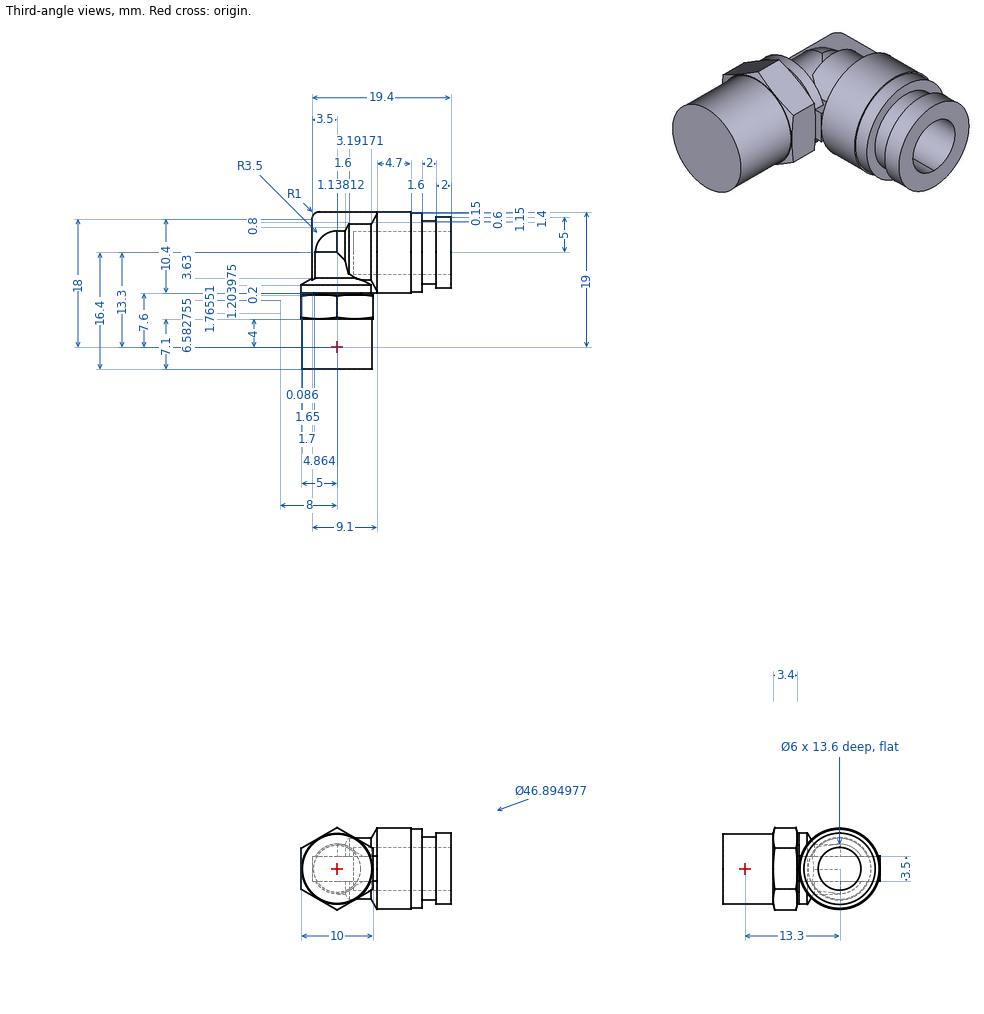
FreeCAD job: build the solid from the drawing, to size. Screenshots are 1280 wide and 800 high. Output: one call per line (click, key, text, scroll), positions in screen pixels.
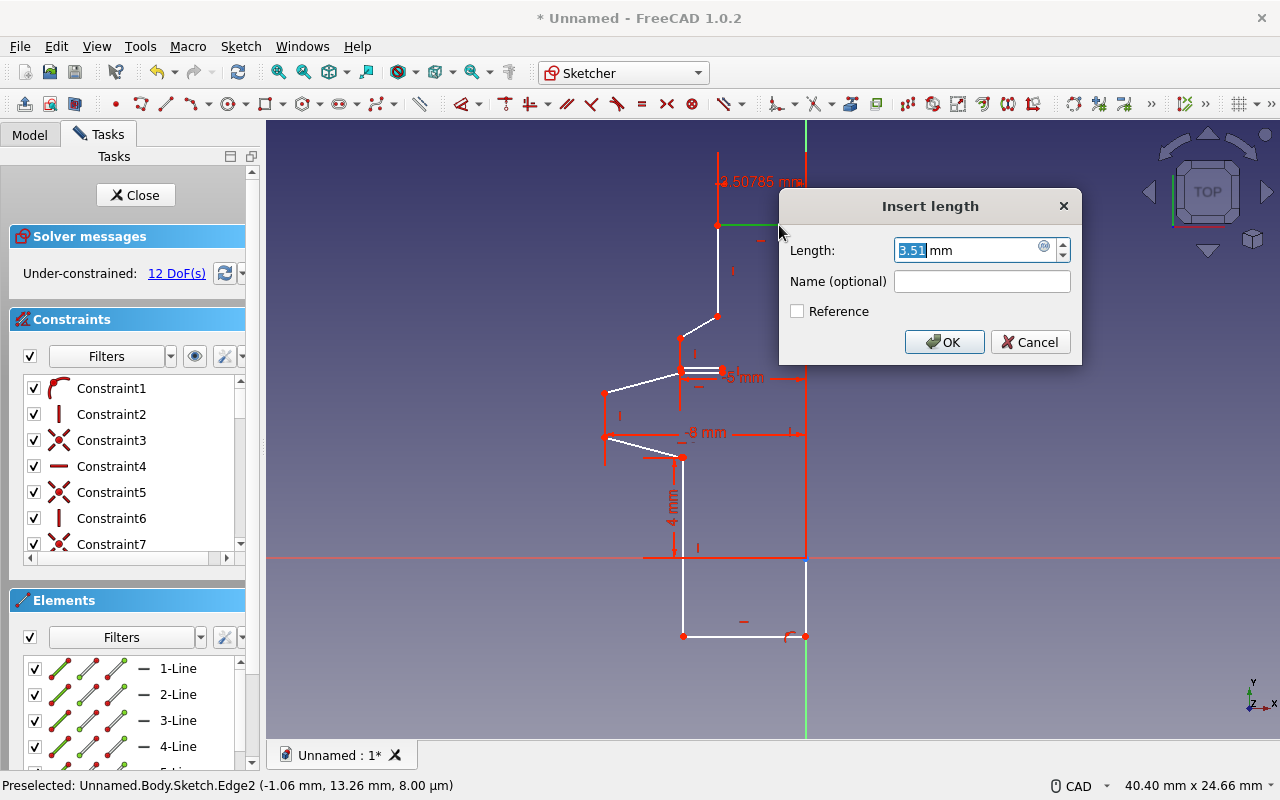
text(3.5)
key(Return)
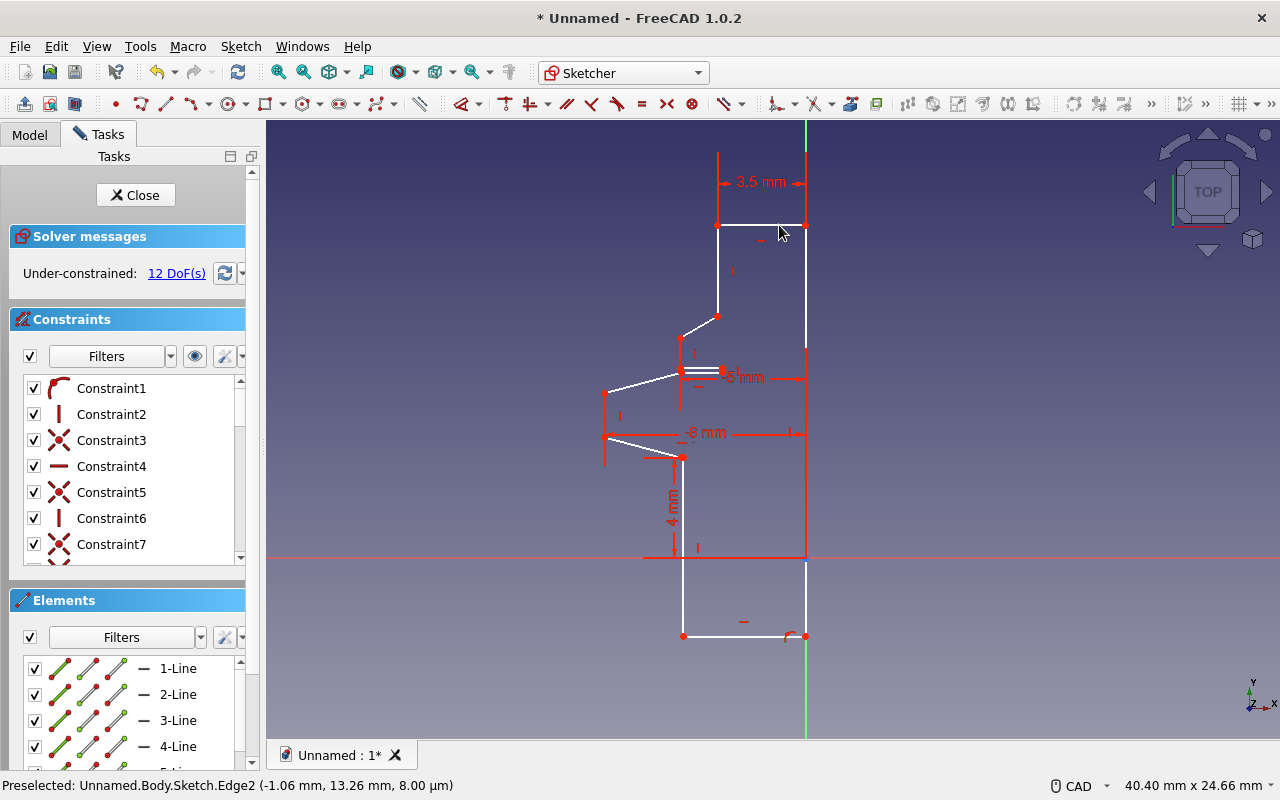
scroll(693, 368, up, 6)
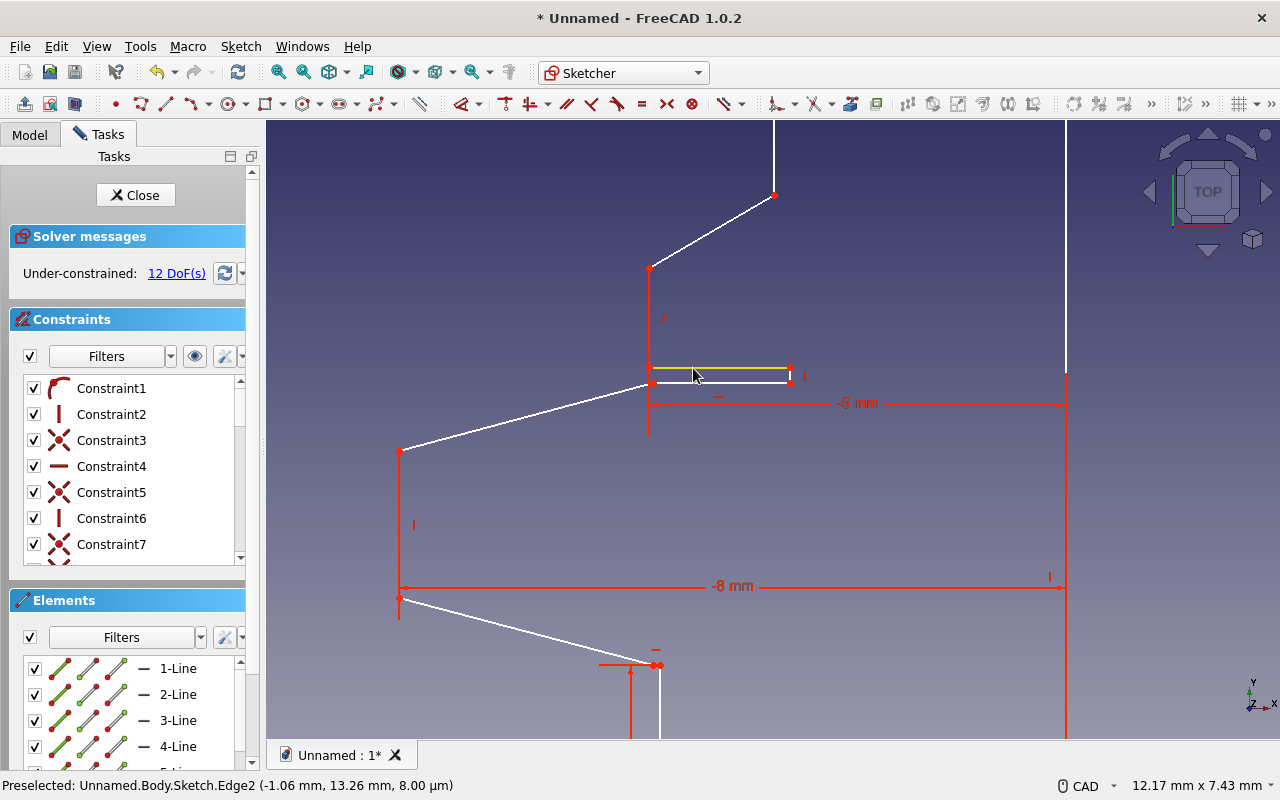
click(692, 368)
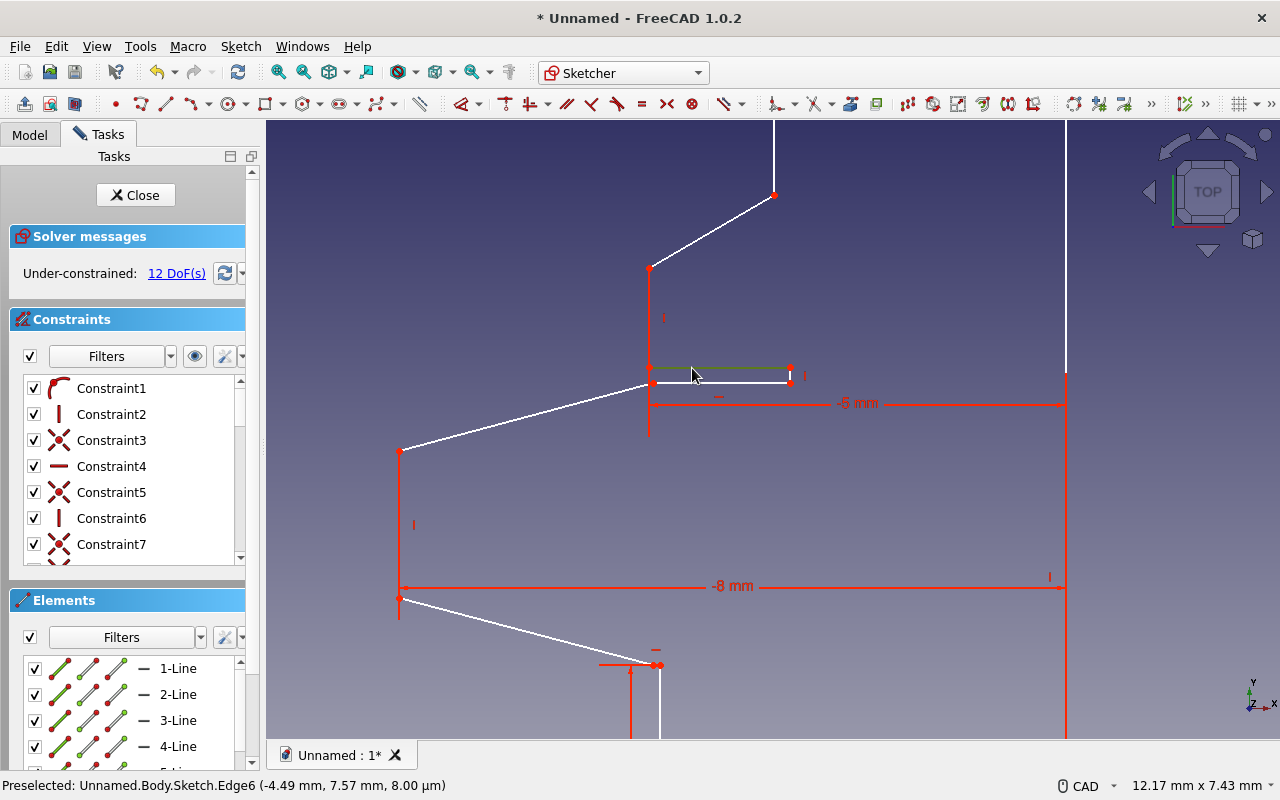
key(l)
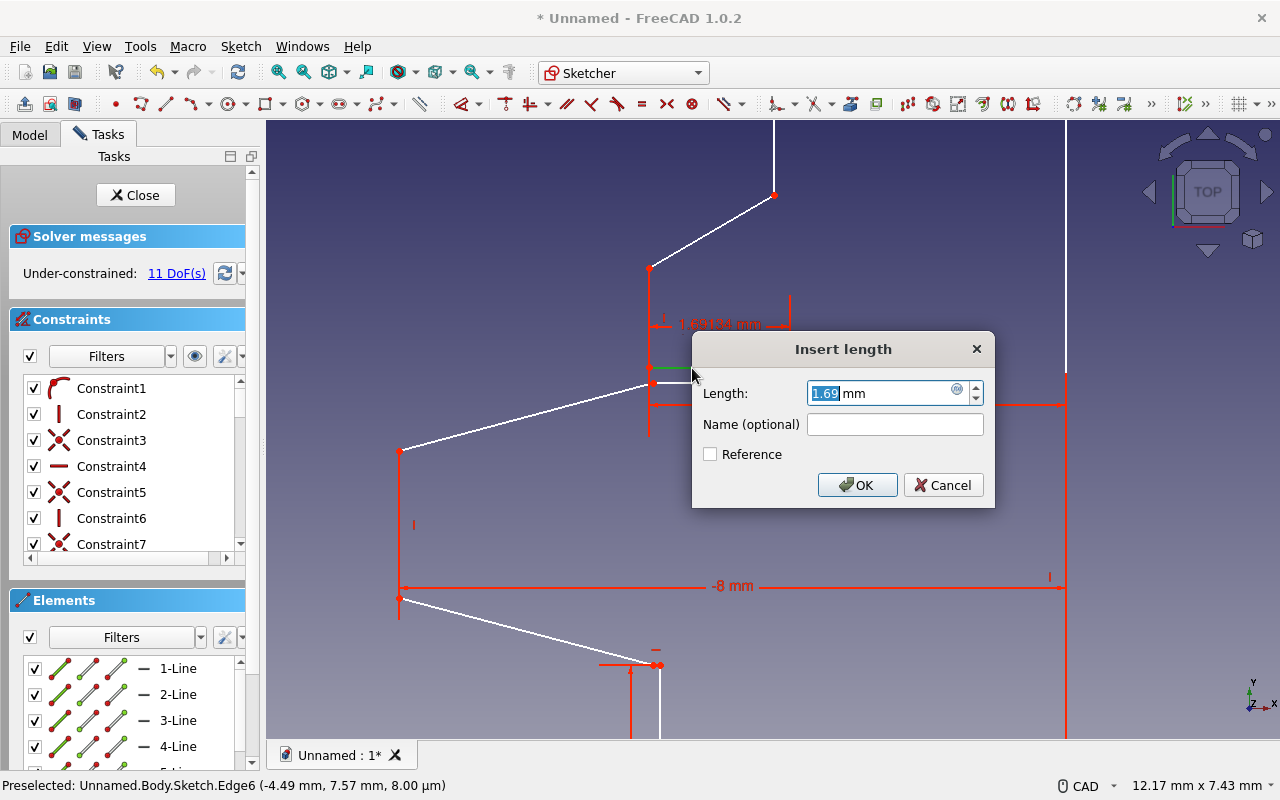
text(1.7)
key(Return)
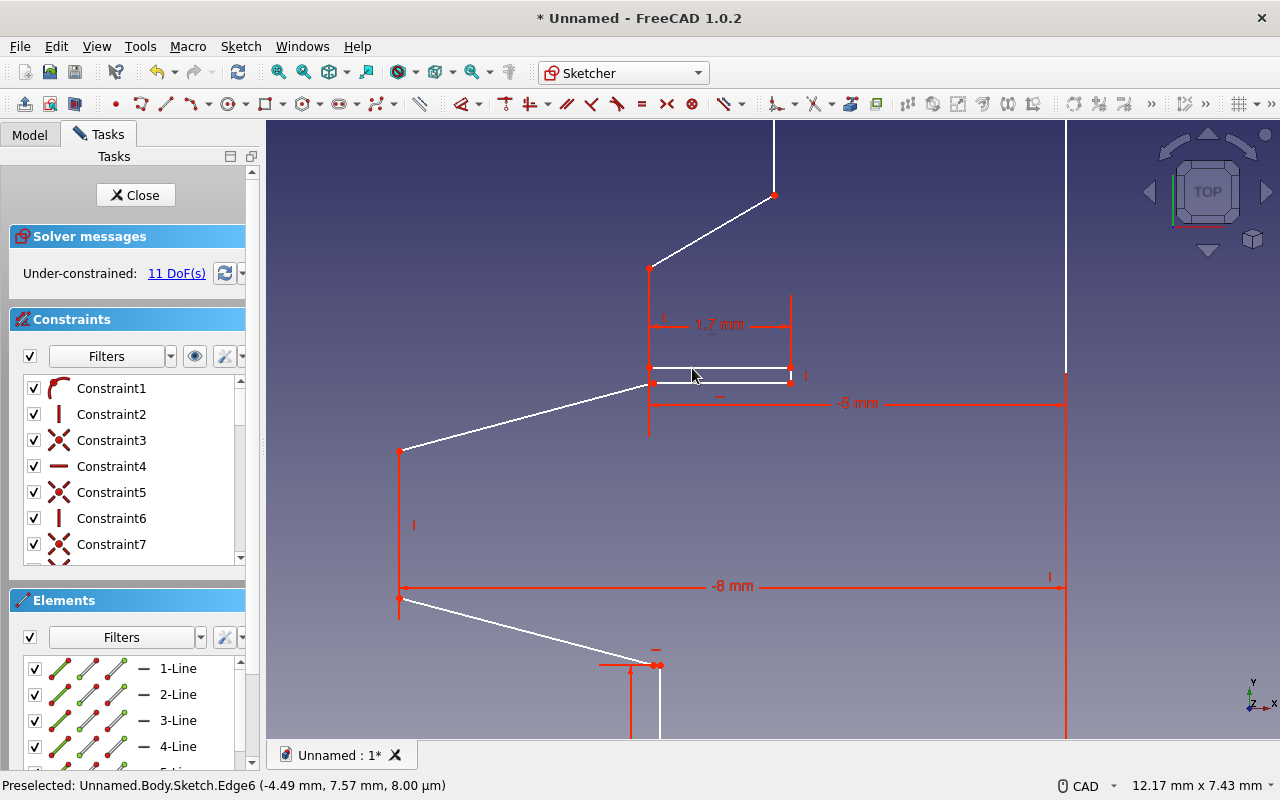
scroll(791, 375, up, 5)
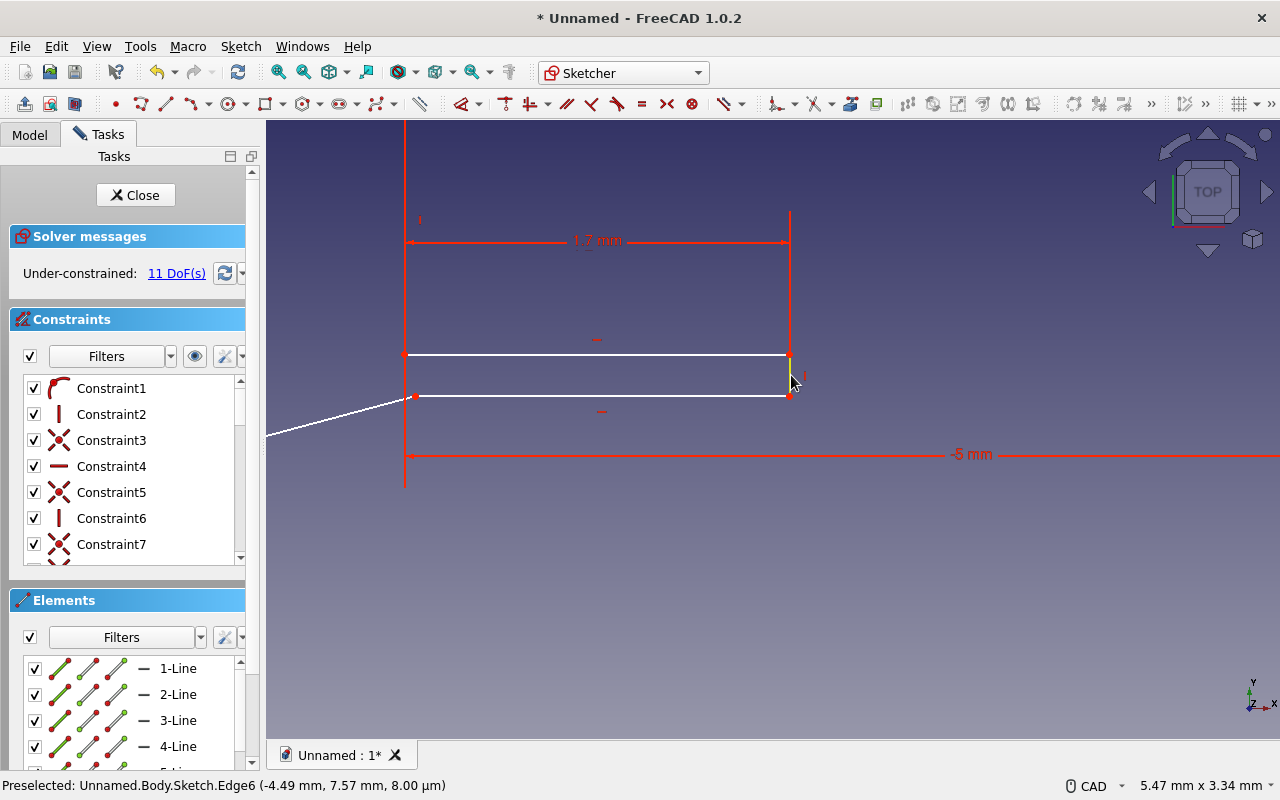
click(790, 375)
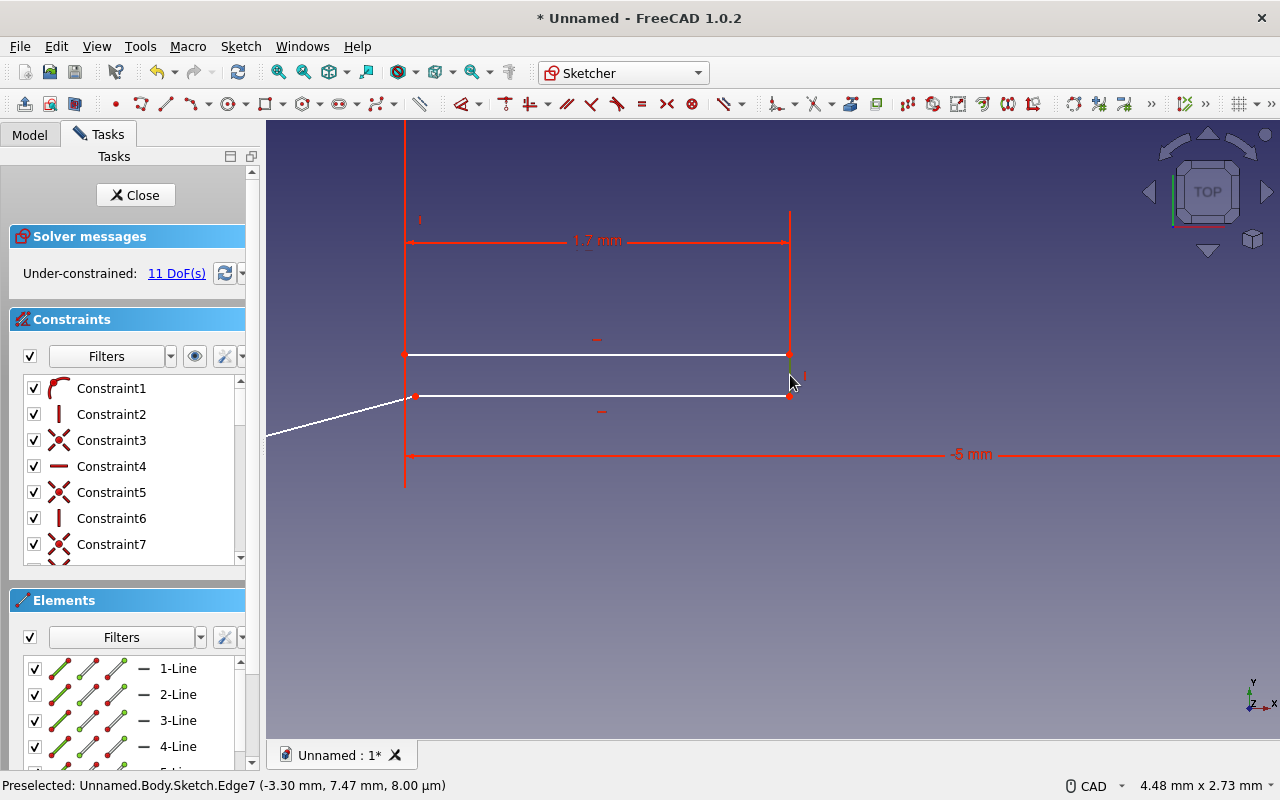
key(i)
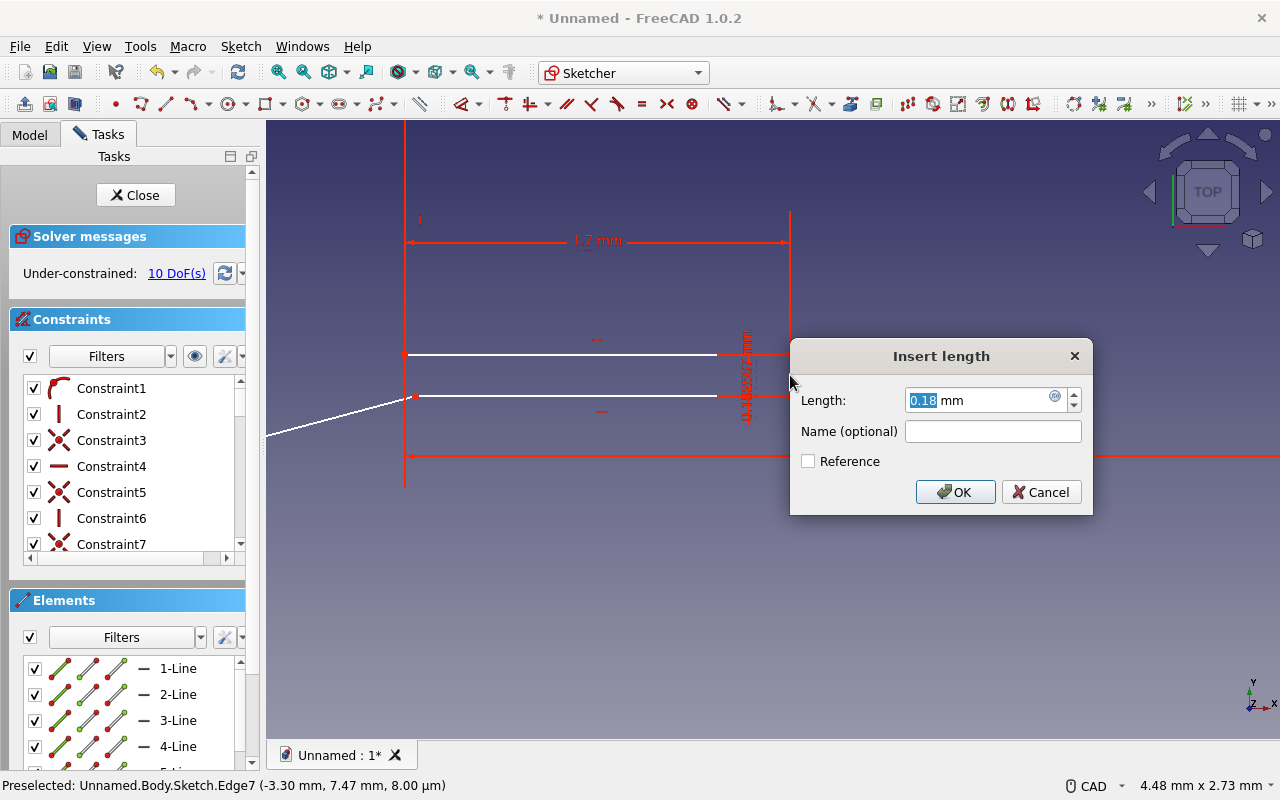
text(0.2)
key(Return)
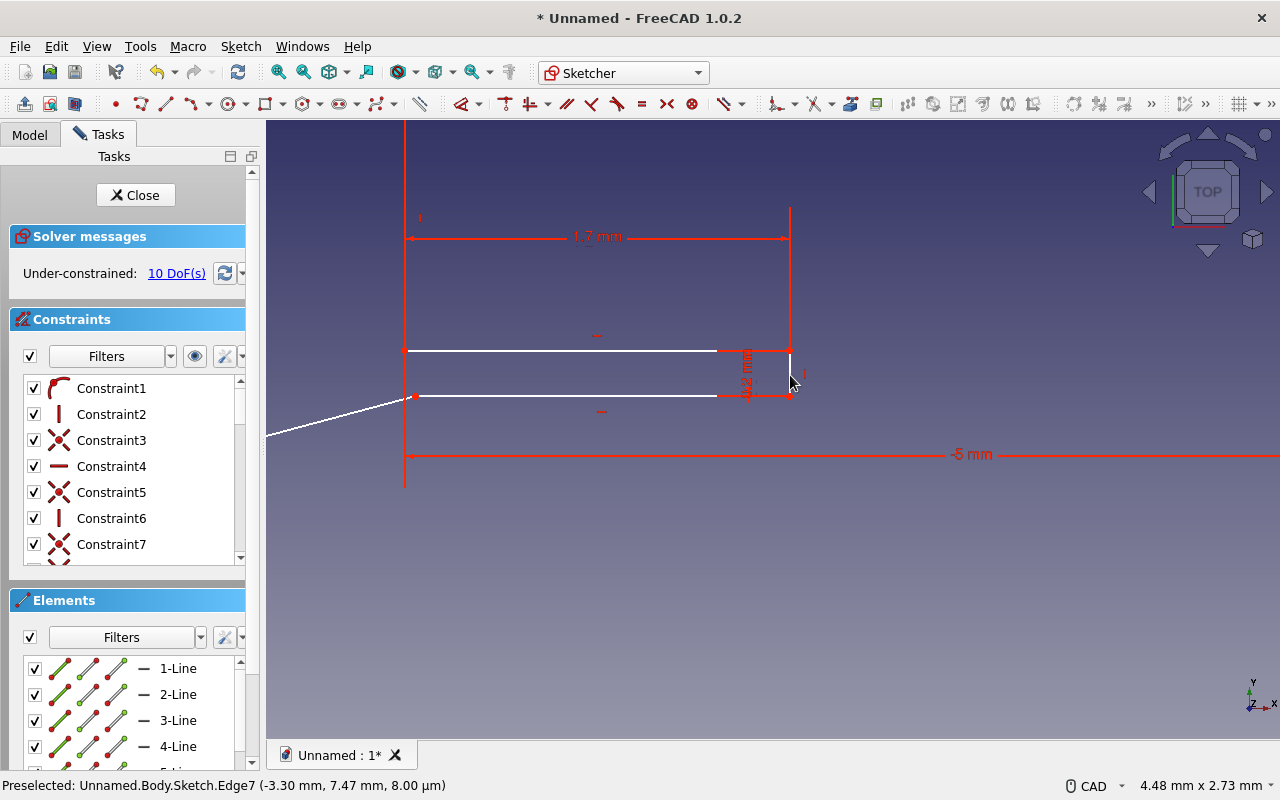
scroll(714, 369, down, 11)